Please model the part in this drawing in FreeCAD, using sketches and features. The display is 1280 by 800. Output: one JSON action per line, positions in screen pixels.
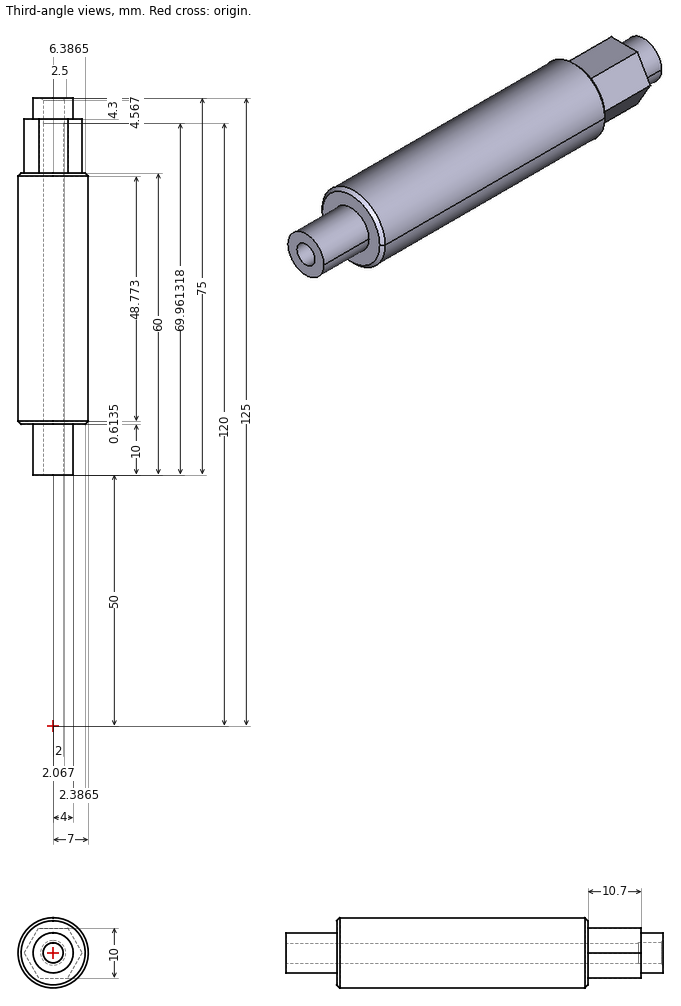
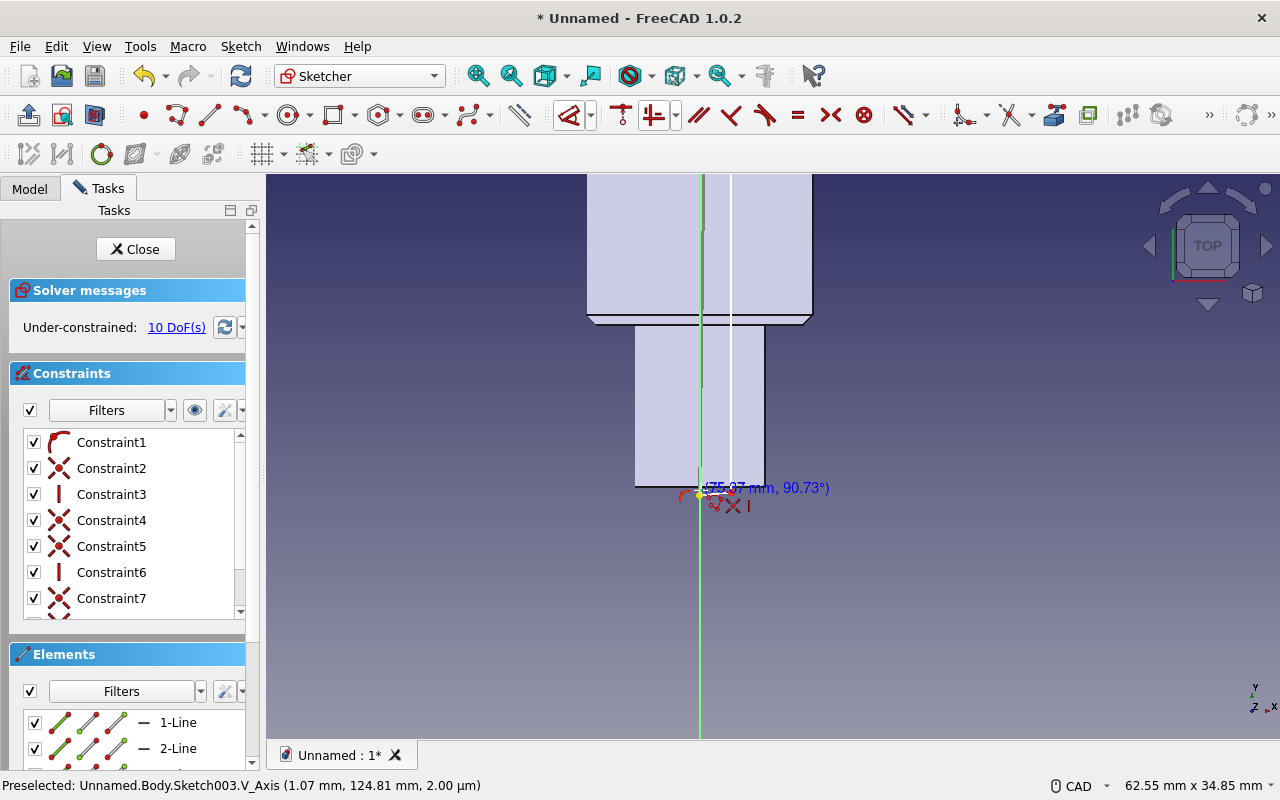
{"action": "left_click", "coordinate": [700, 496]}
{"action": "key", "text": "Escape"}
{"action": "key", "text": "Escape"}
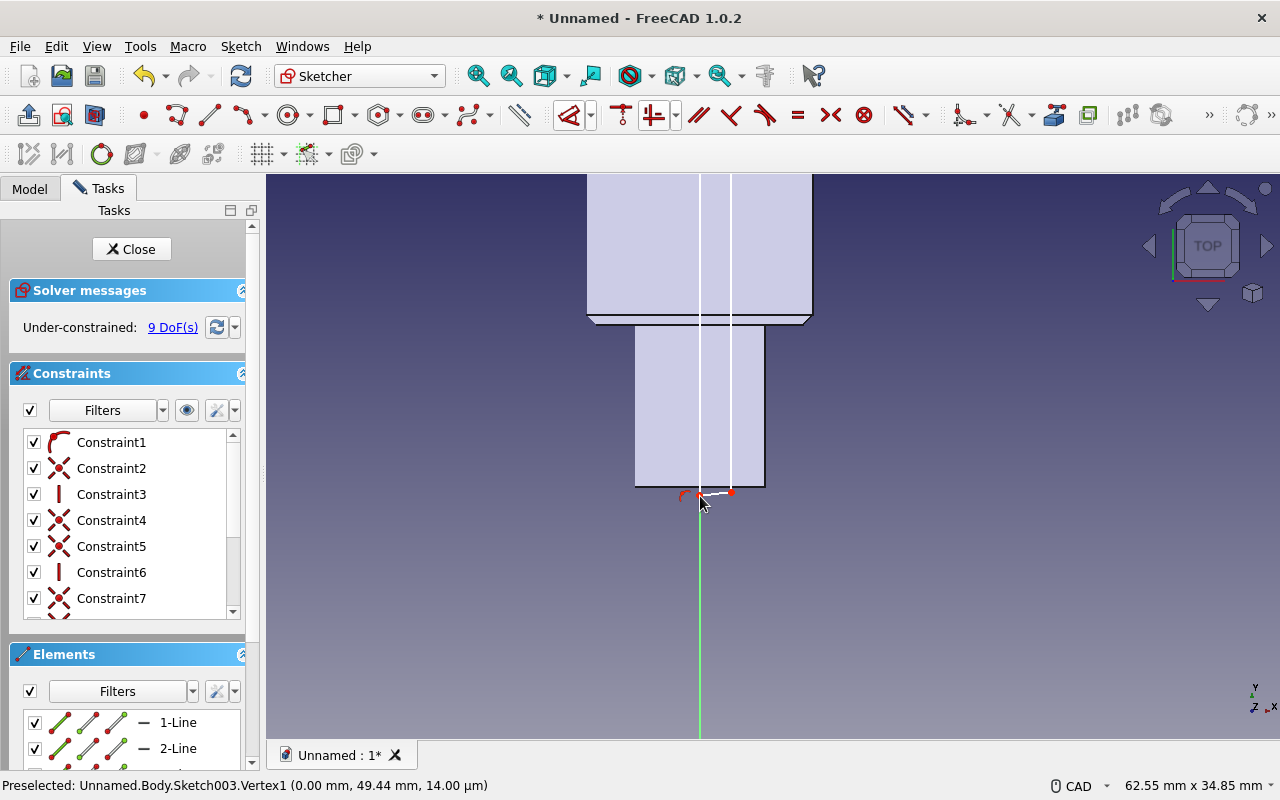
{"action": "scroll", "coordinate": [709, 495], "scroll_direction": "up", "scroll_amount": 2}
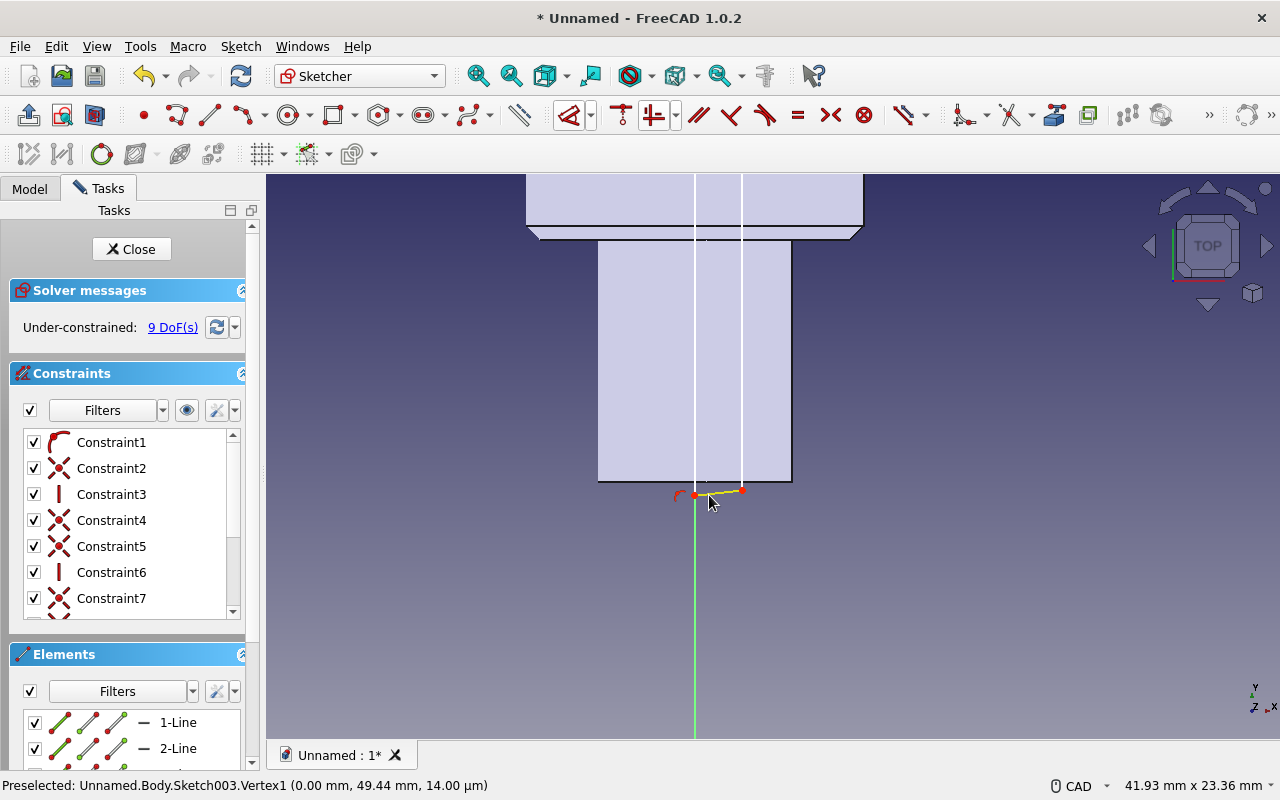
{"action": "left_click", "coordinate": [709, 494]}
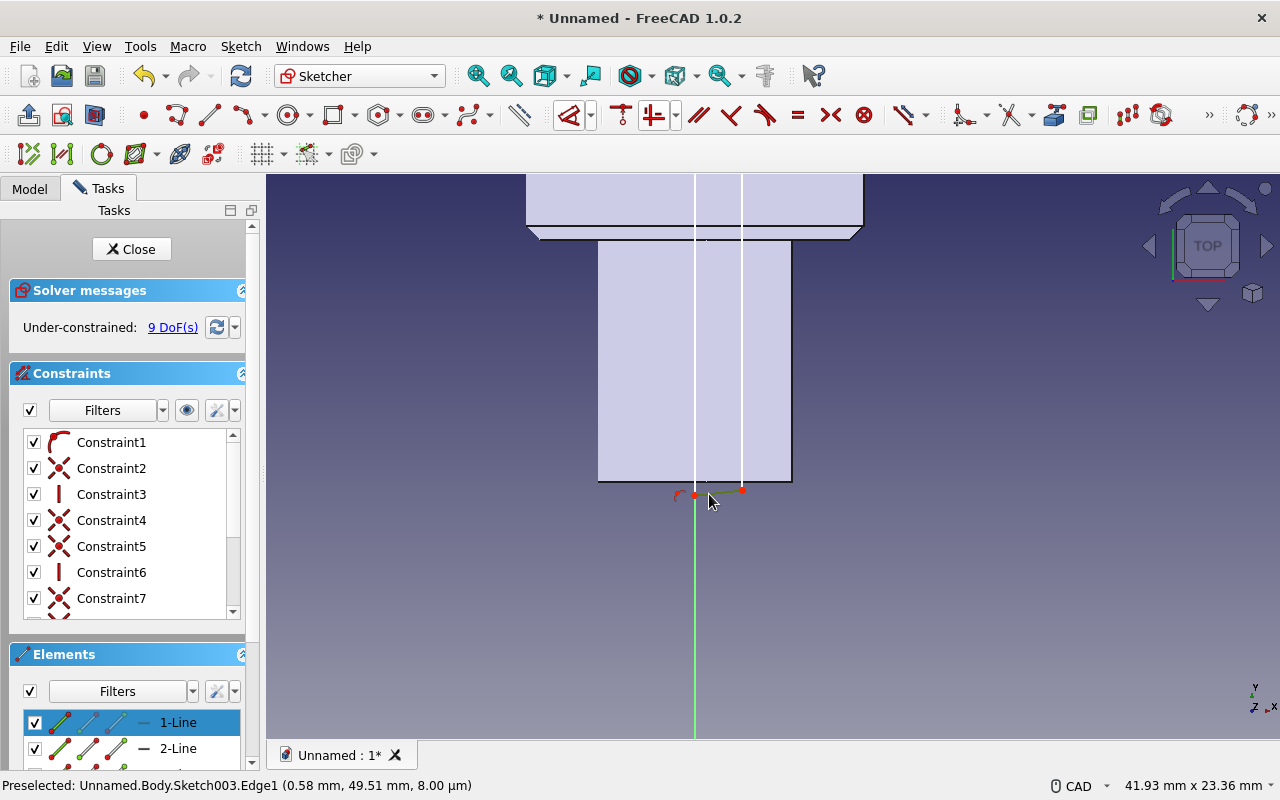
{"action": "key", "text": "h"}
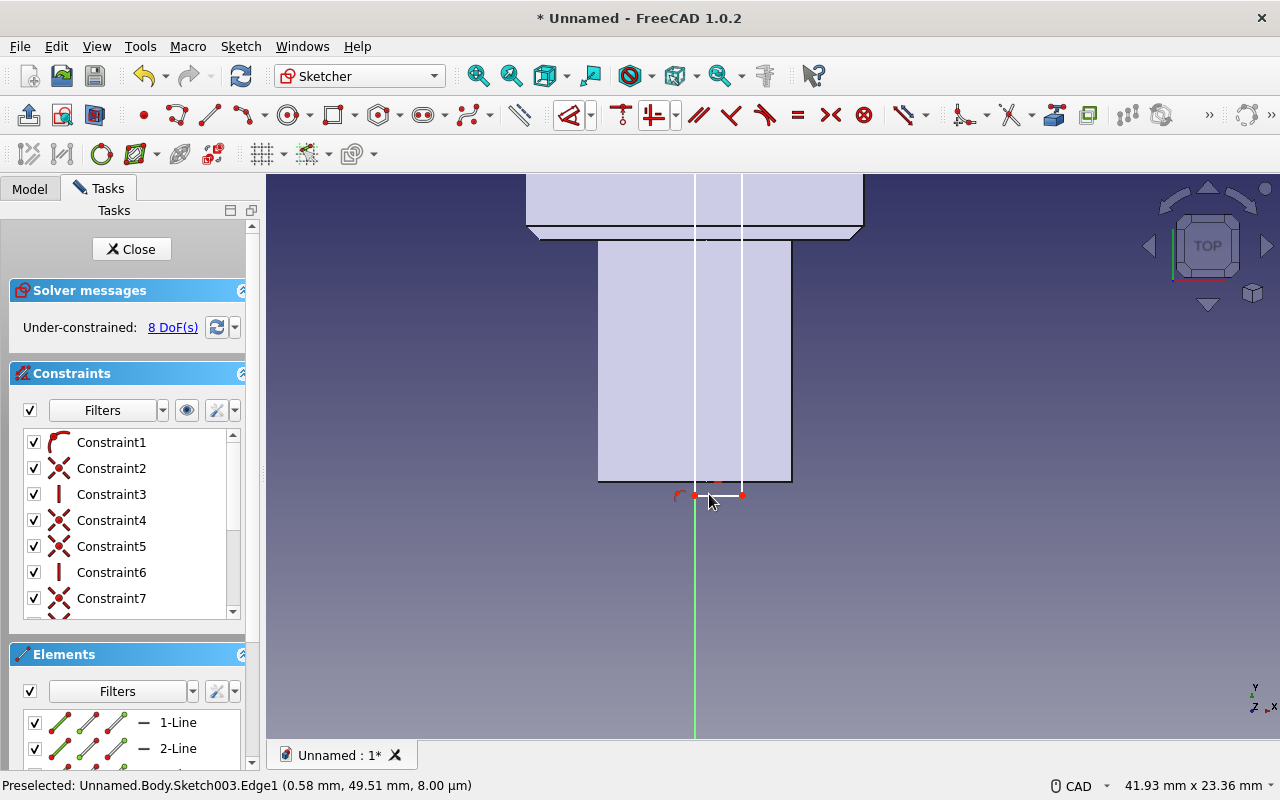
{"action": "left_click", "coordinate": [709, 496]}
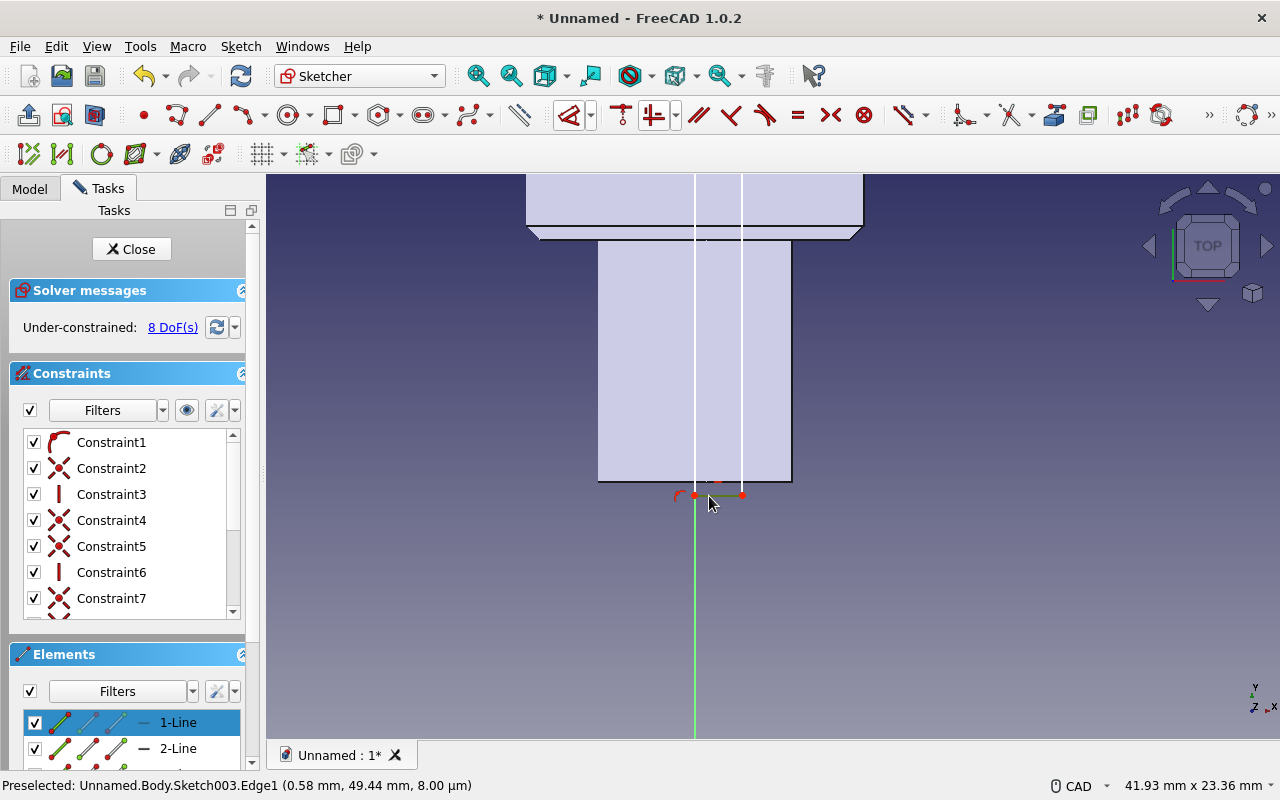
{"action": "key", "text": "l"}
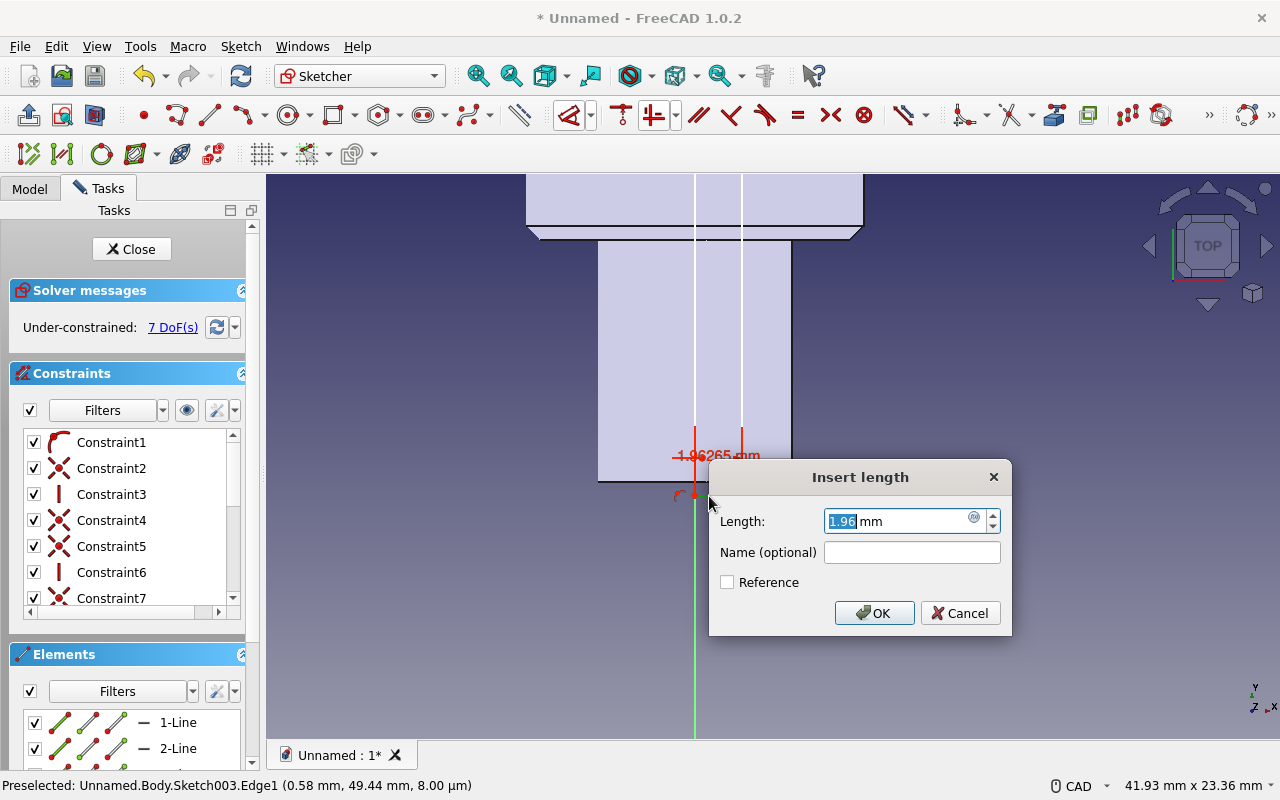
{"action": "type", "text": "2"}
{"action": "key", "text": "Return"}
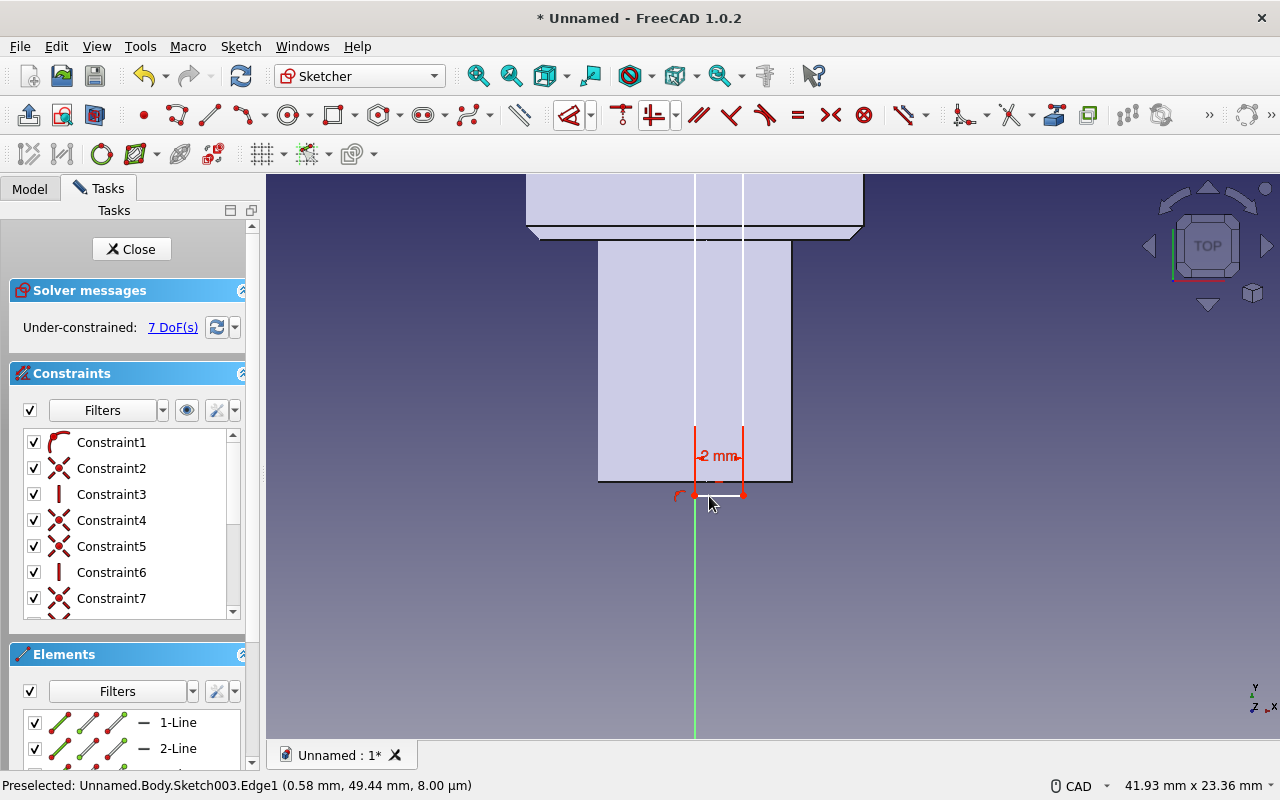
{"action": "scroll", "coordinate": [702, 491], "scroll_direction": "down", "scroll_amount": 11}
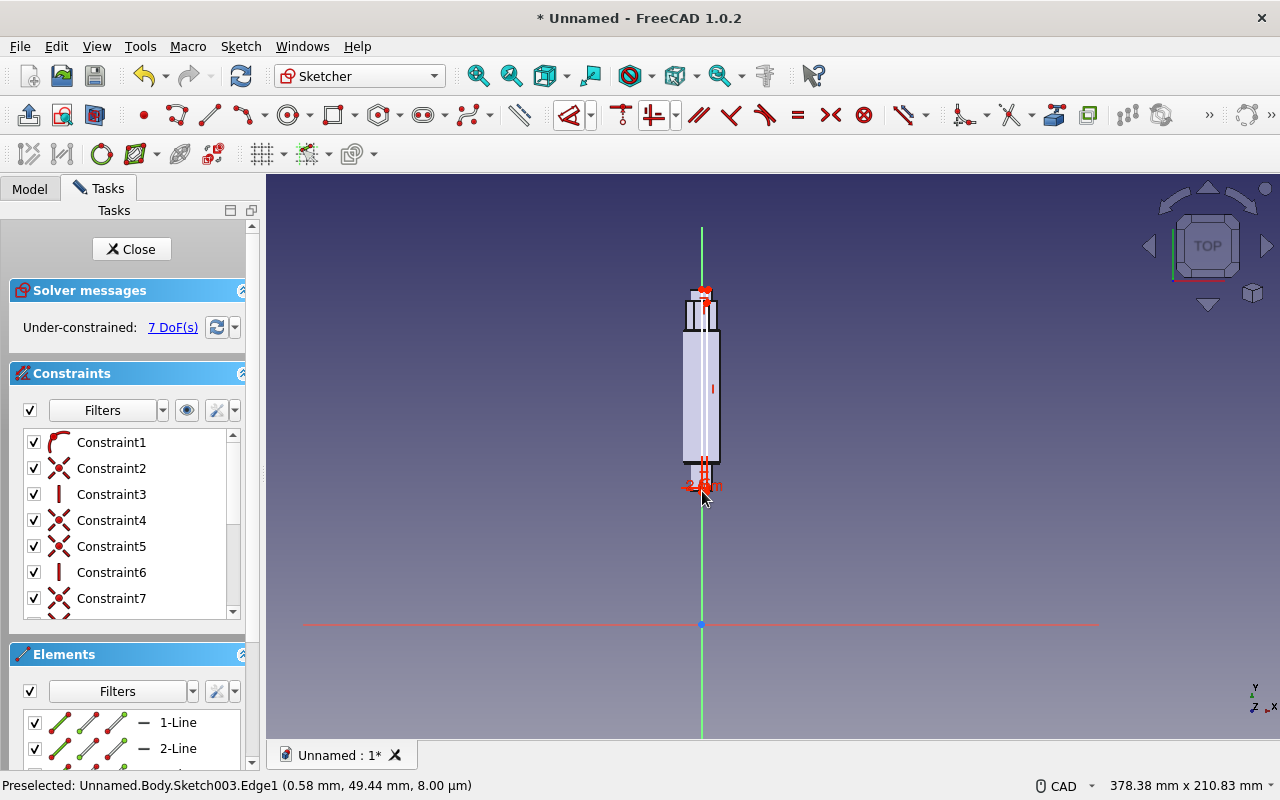
{"action": "scroll", "coordinate": [702, 350], "scroll_direction": "up", "scroll_amount": 5}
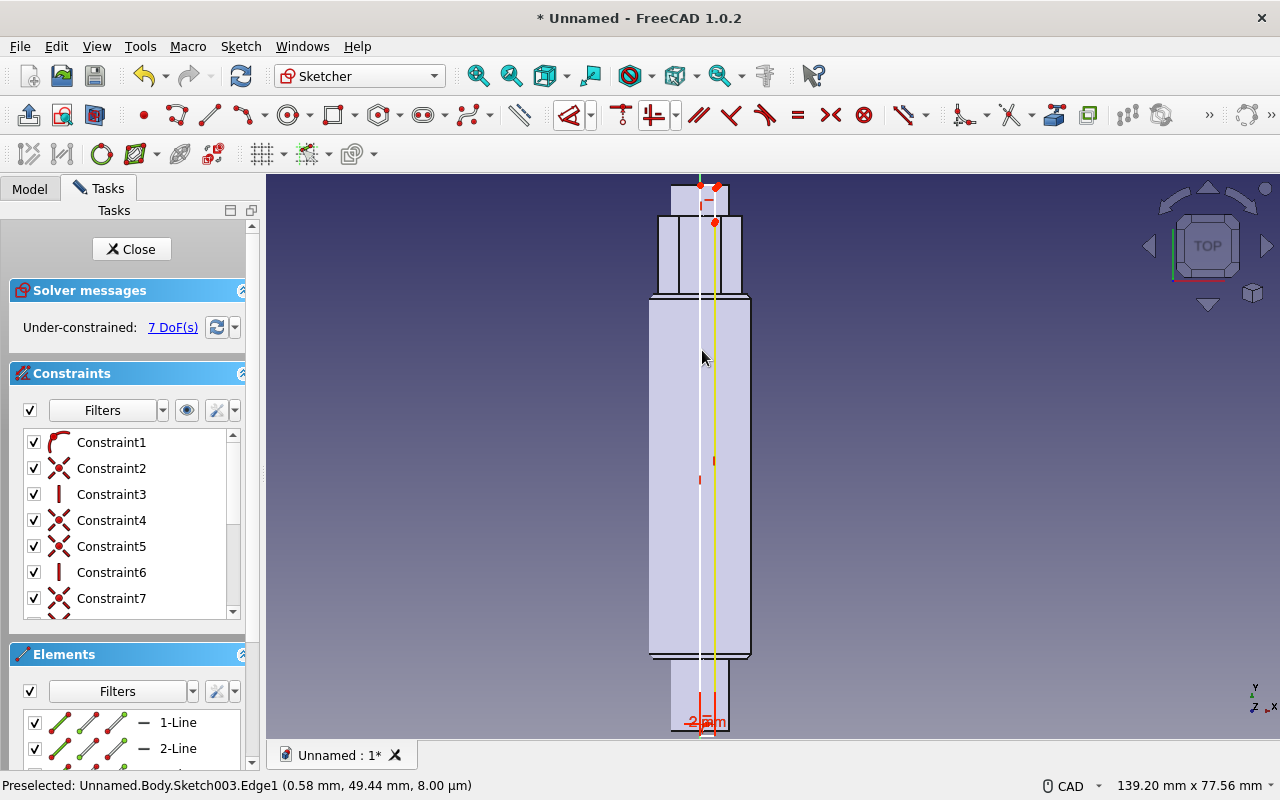
{"action": "left_click", "coordinate": [700, 350]}